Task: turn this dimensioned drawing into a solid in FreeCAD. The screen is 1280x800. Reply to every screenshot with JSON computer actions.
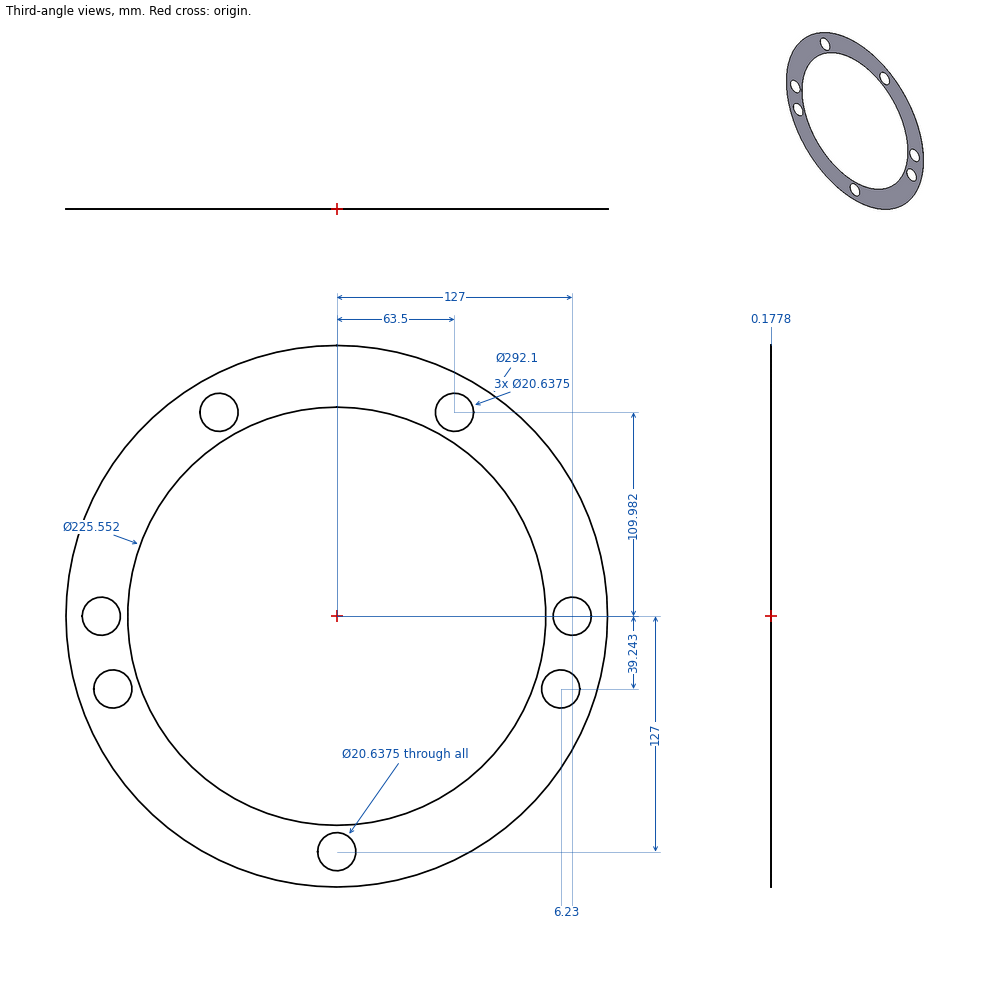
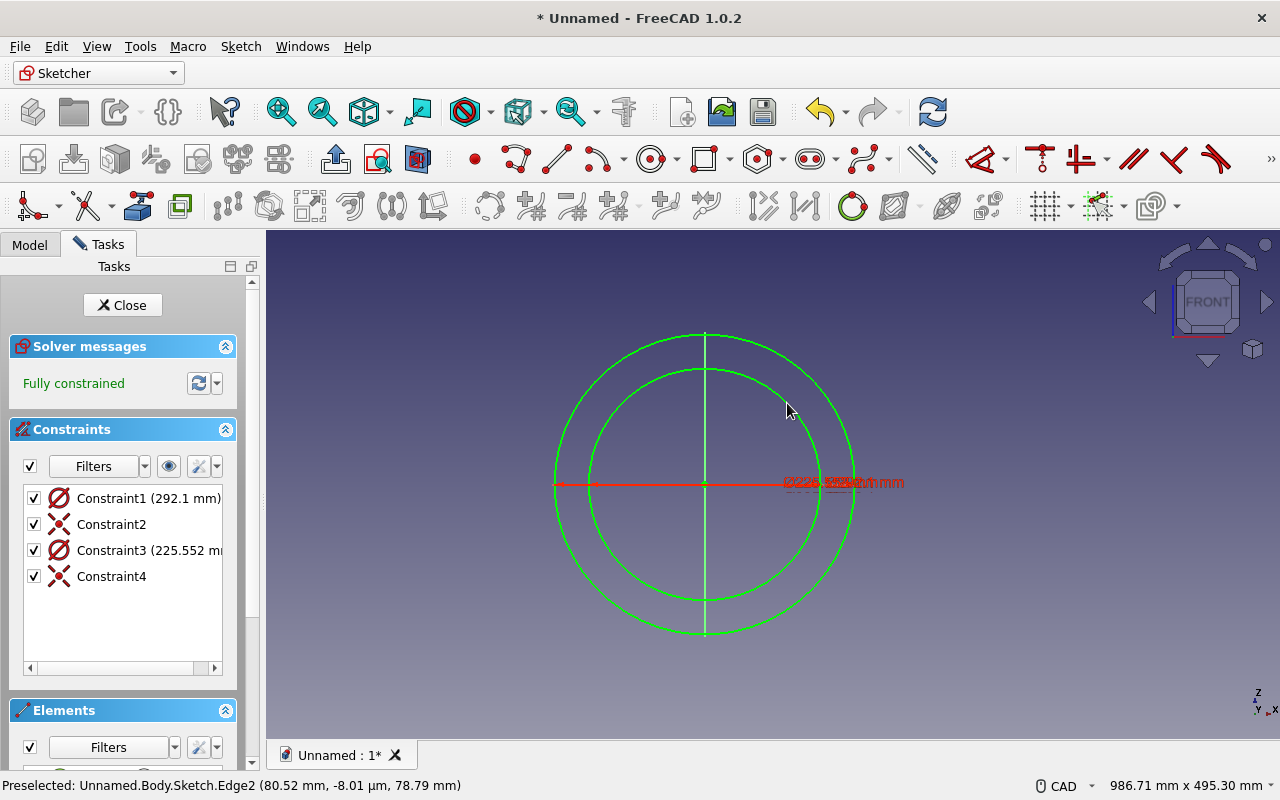
{"action": "left_click", "coordinate": [123, 305]}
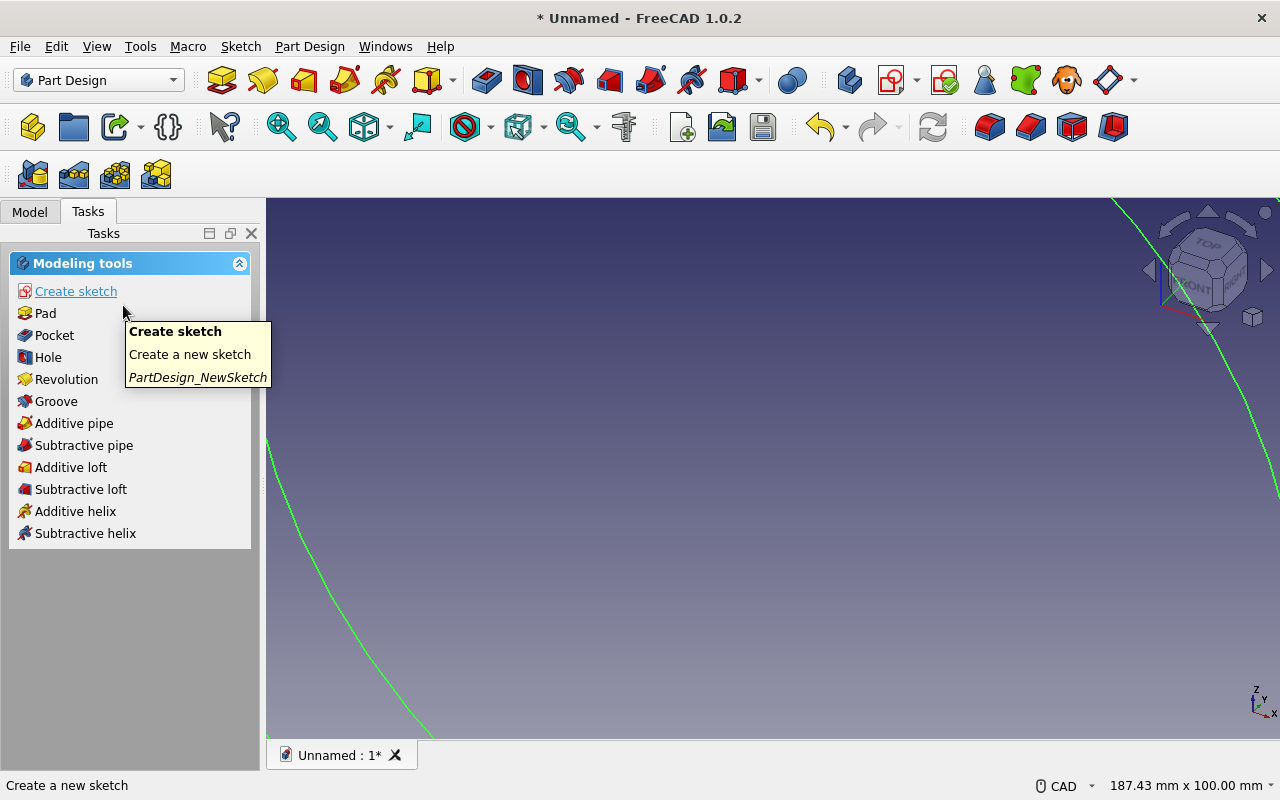
{"action": "left_click", "coordinate": [222, 80]}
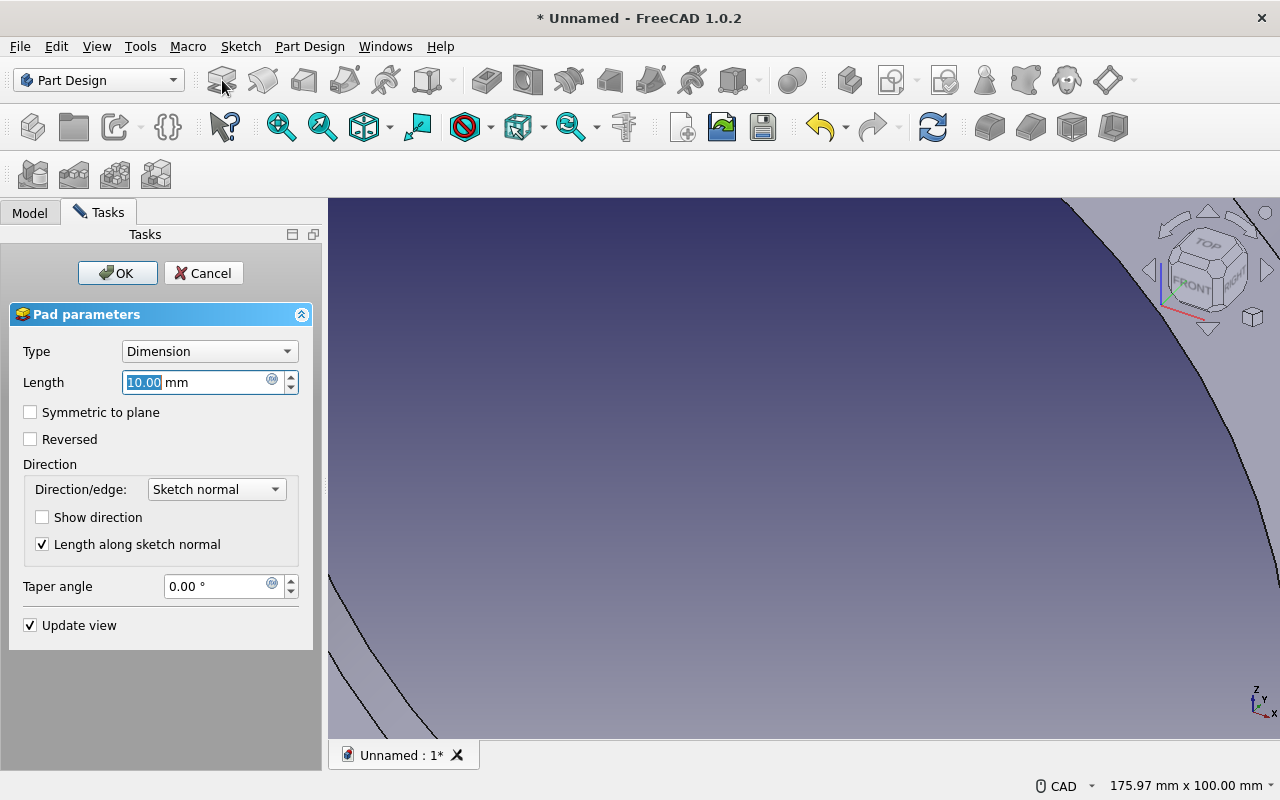
{"action": "type", "text": "0.1778"}
{"action": "key", "text": "Tab"}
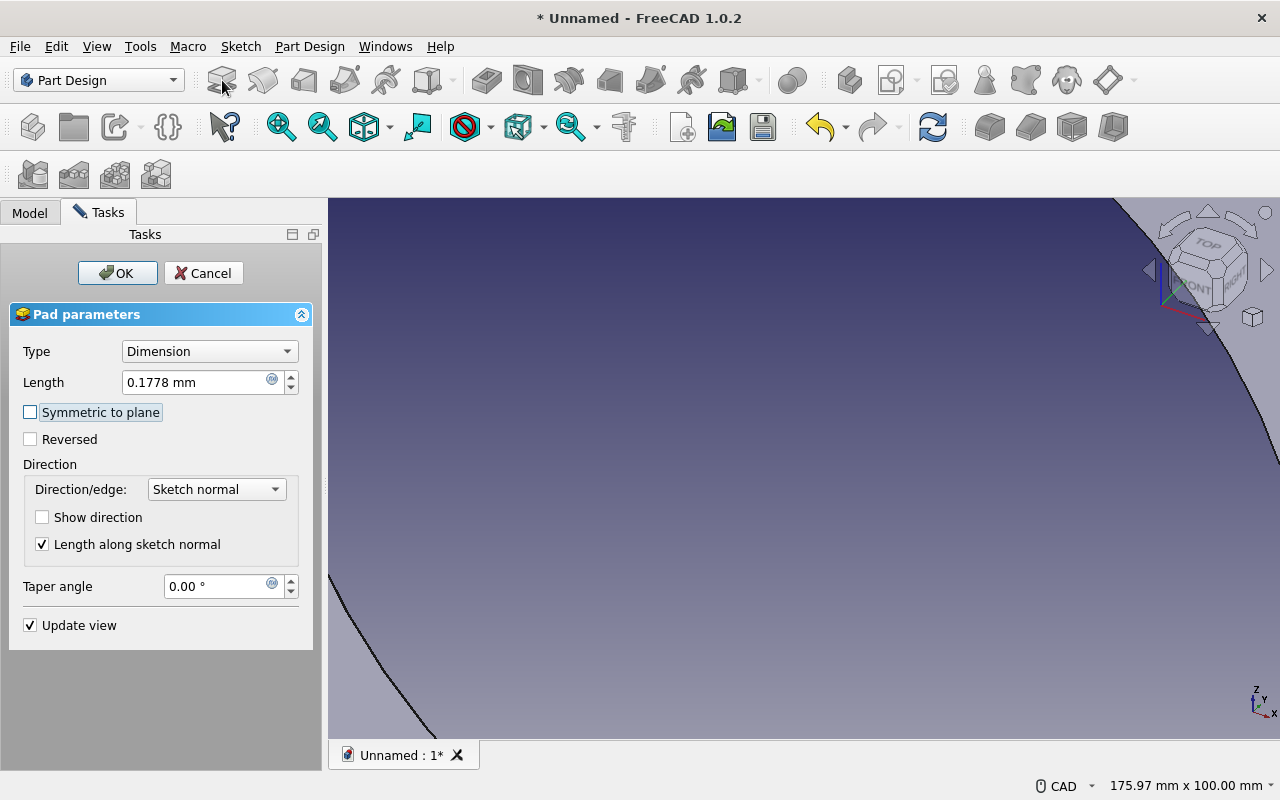
{"action": "left_click", "coordinate": [31, 439]}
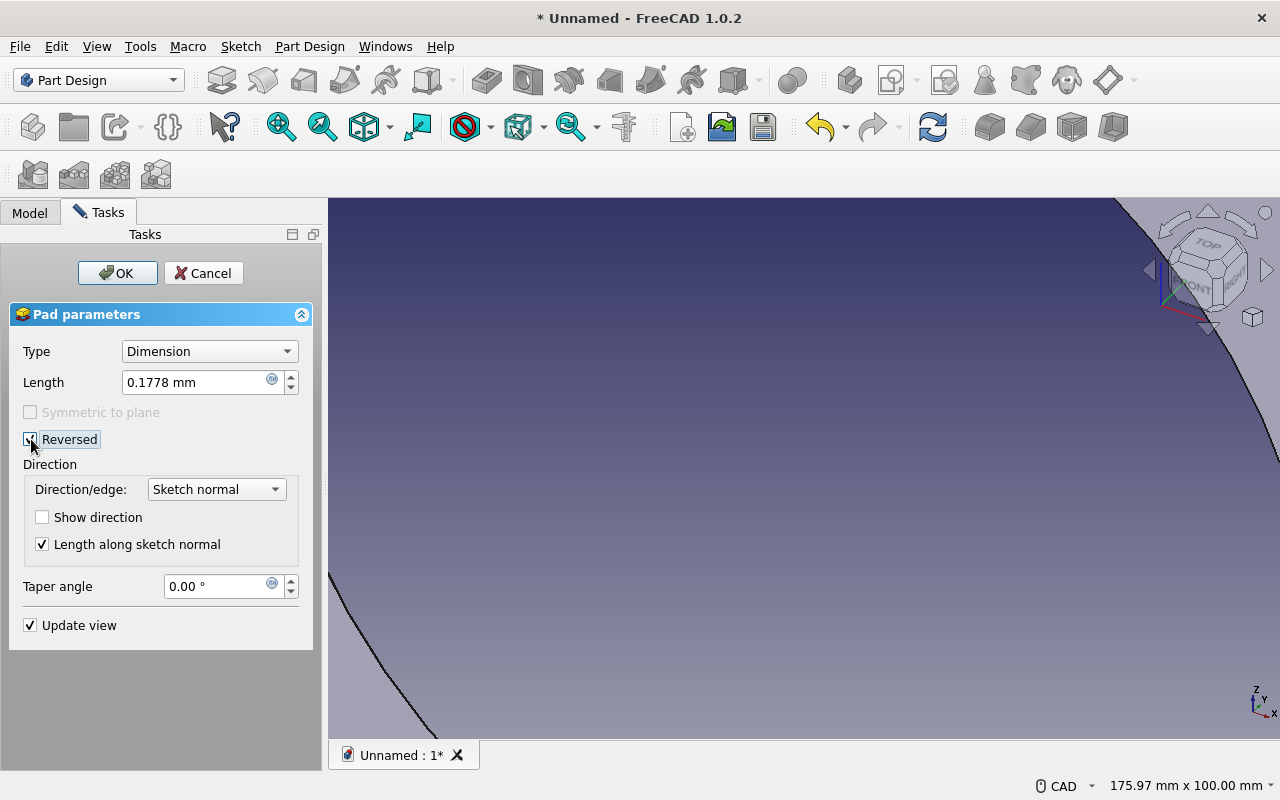
{"action": "left_click", "coordinate": [118, 273]}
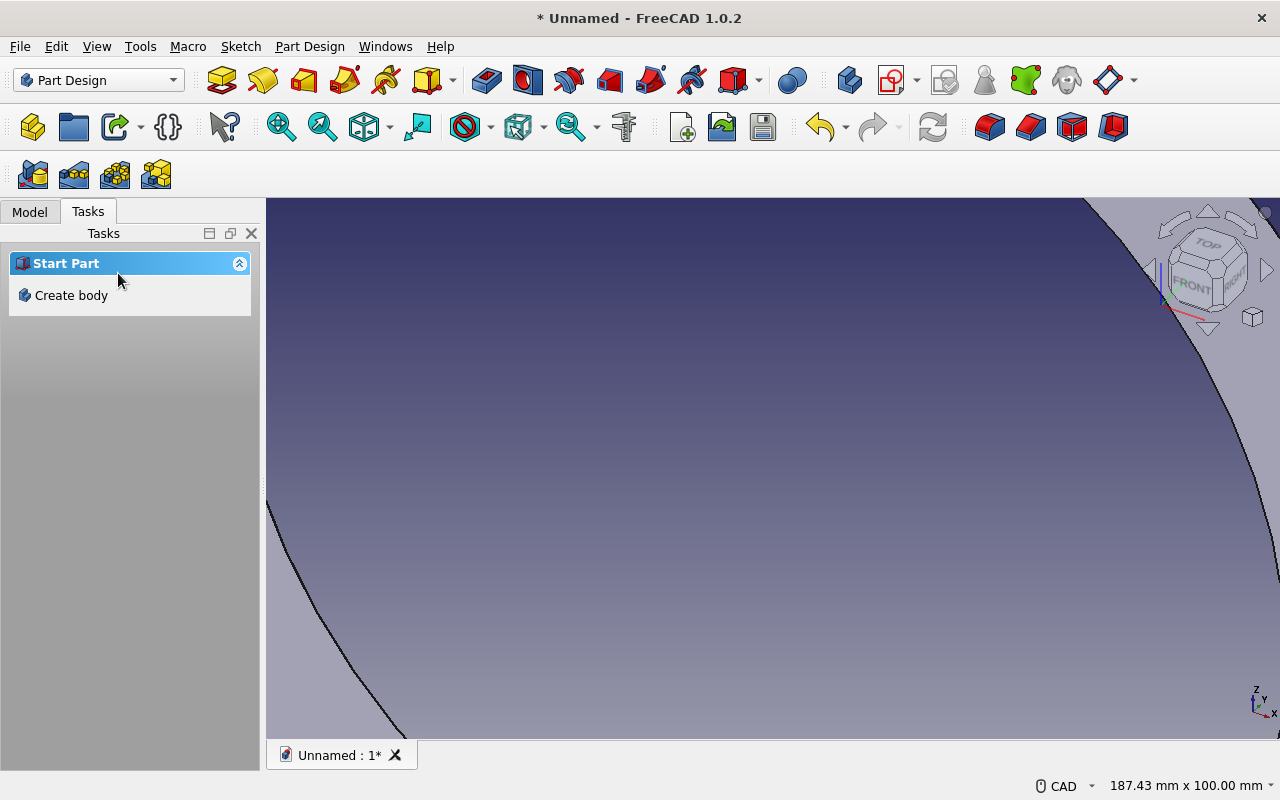
{"action": "left_click", "coordinate": [282, 128]}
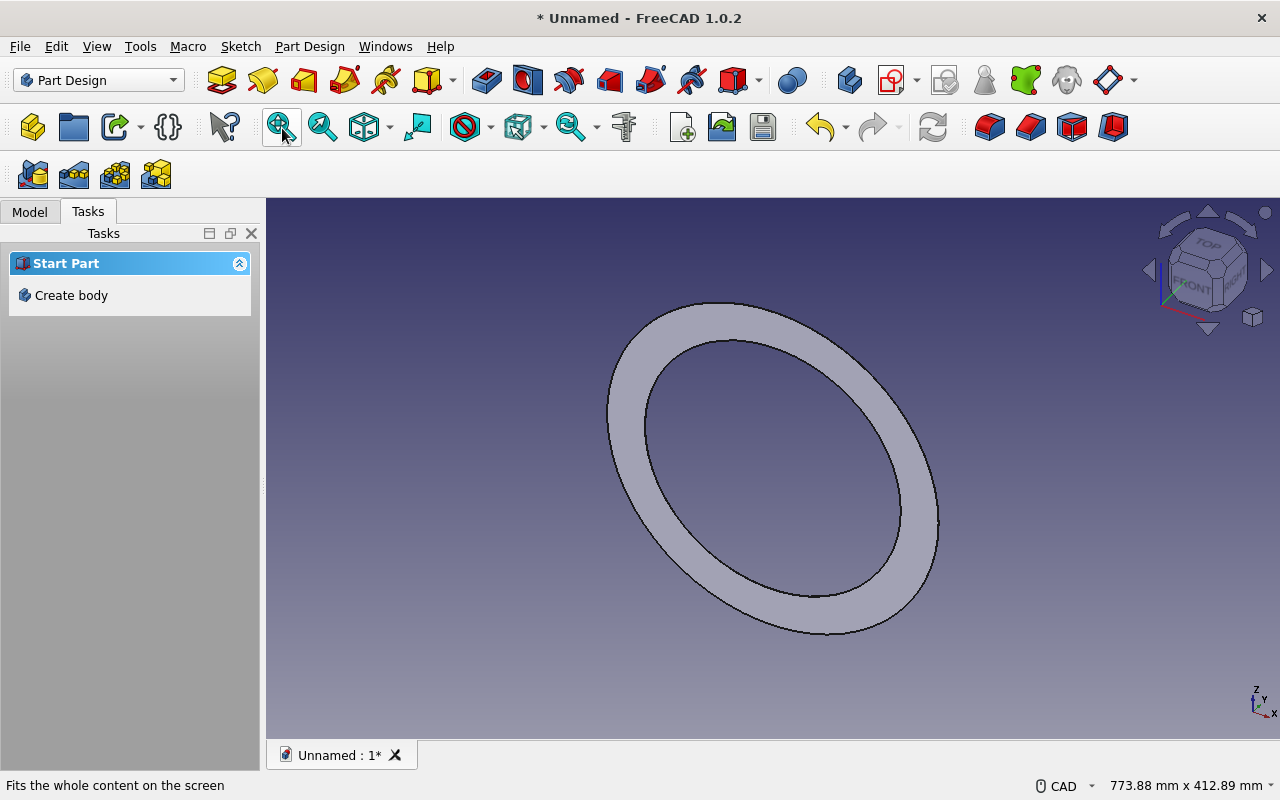
{"action": "key", "text": "4"}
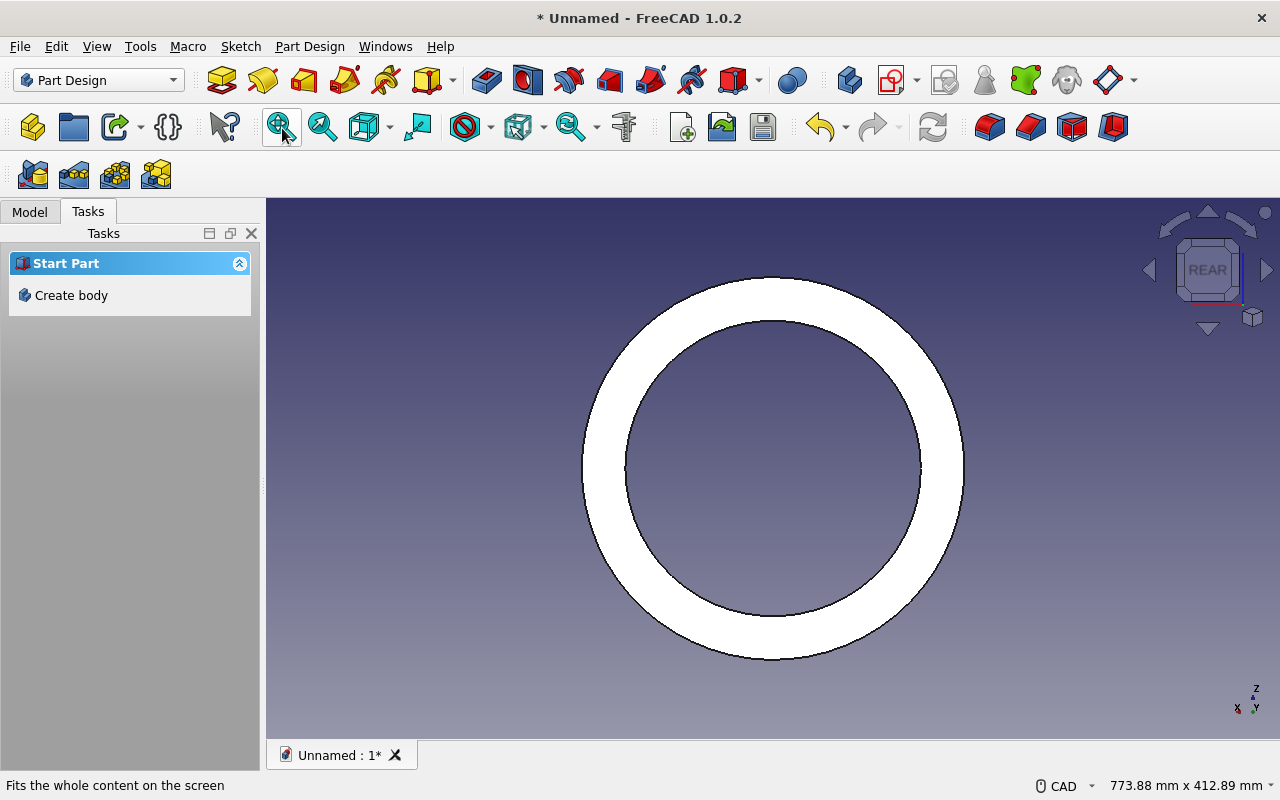
{"action": "left_click", "coordinate": [718, 632]}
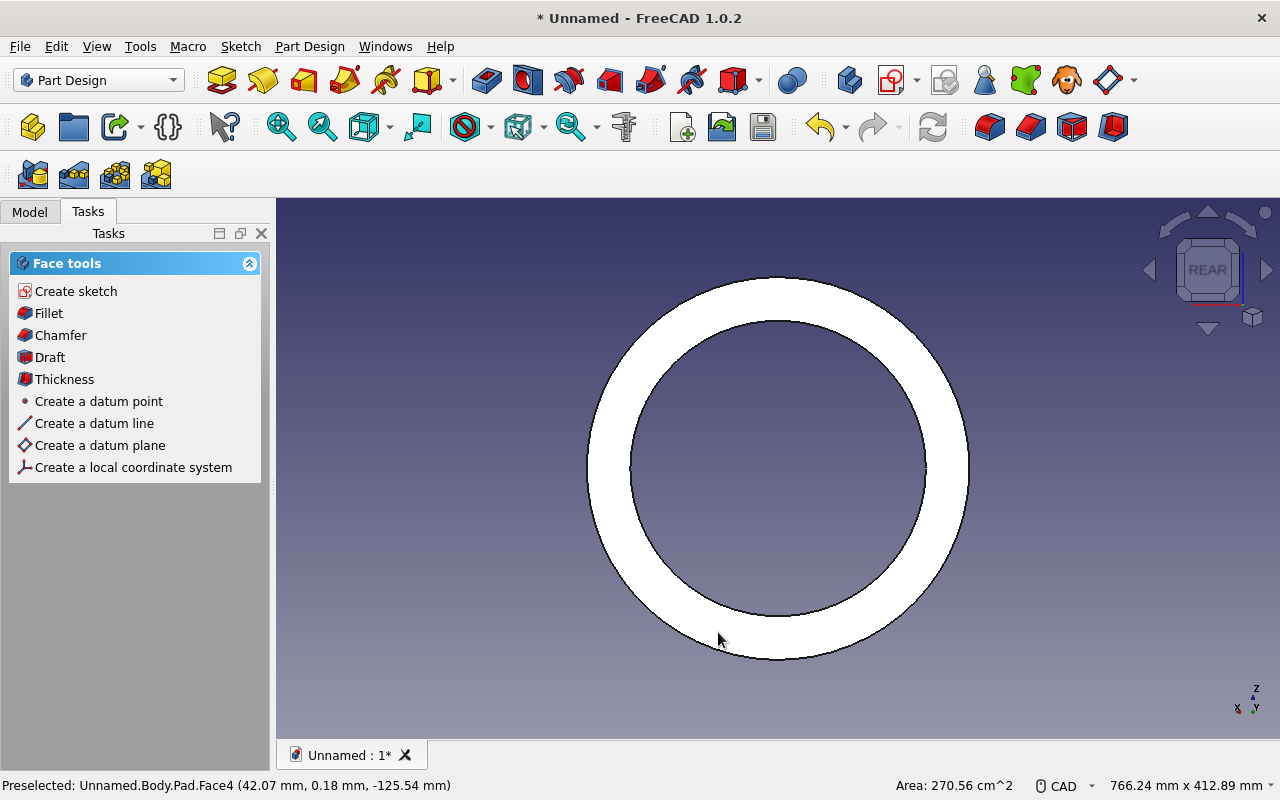
{"action": "left_click", "coordinate": [890, 80]}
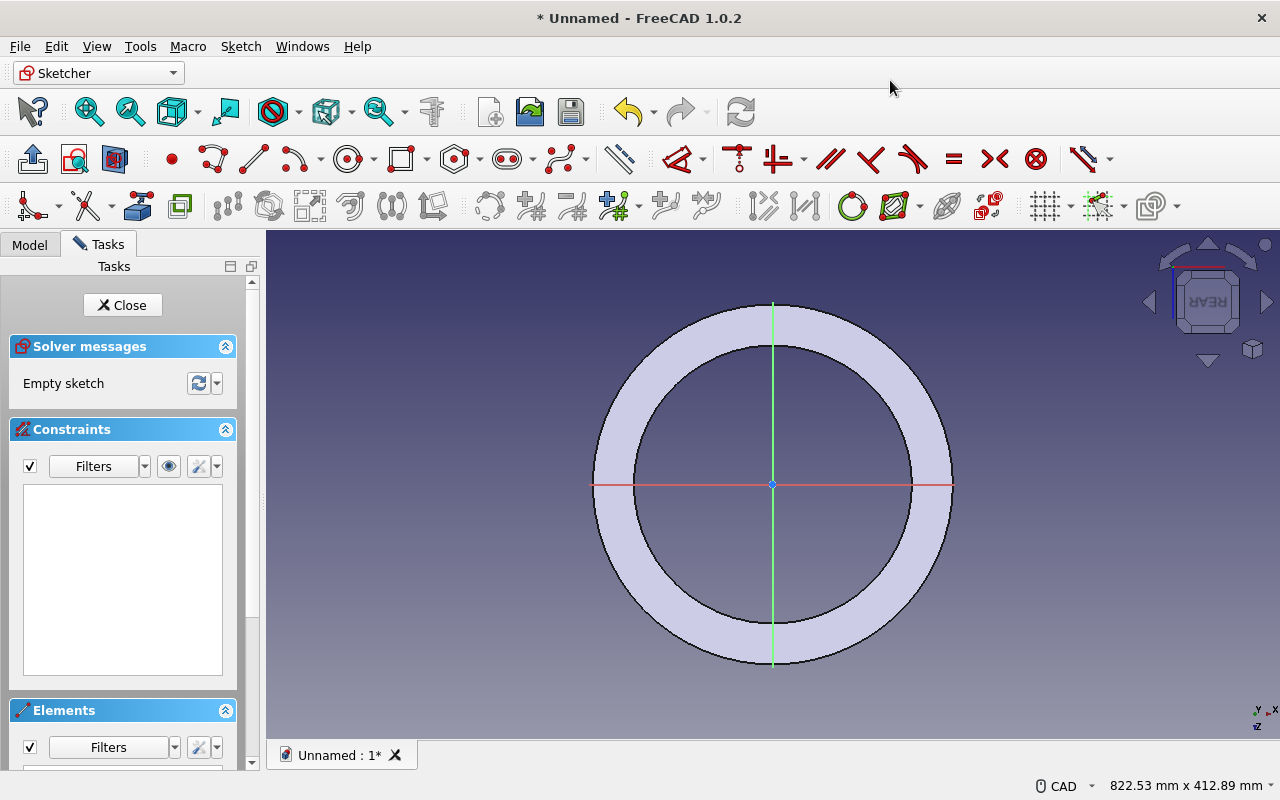
{"action": "scroll", "coordinate": [778, 315], "scroll_direction": "up", "scroll_amount": 13}